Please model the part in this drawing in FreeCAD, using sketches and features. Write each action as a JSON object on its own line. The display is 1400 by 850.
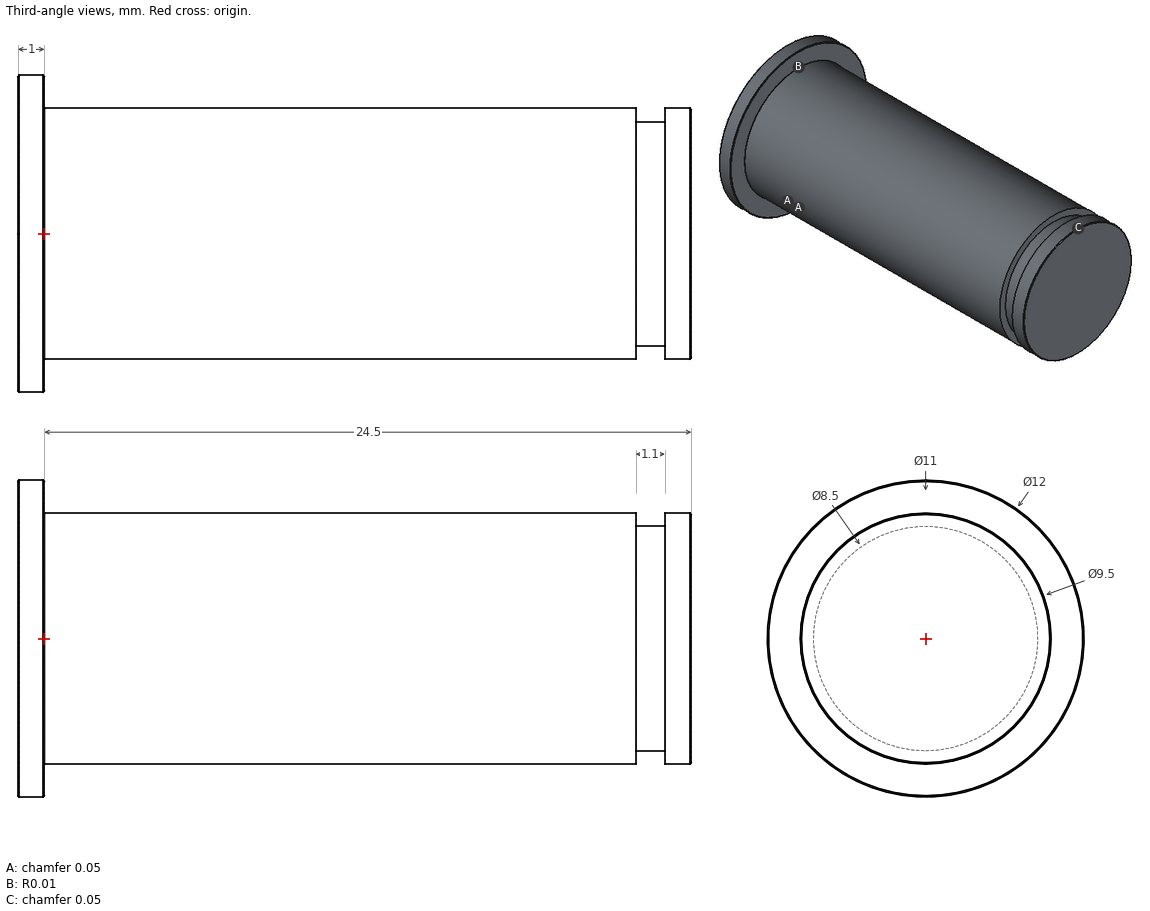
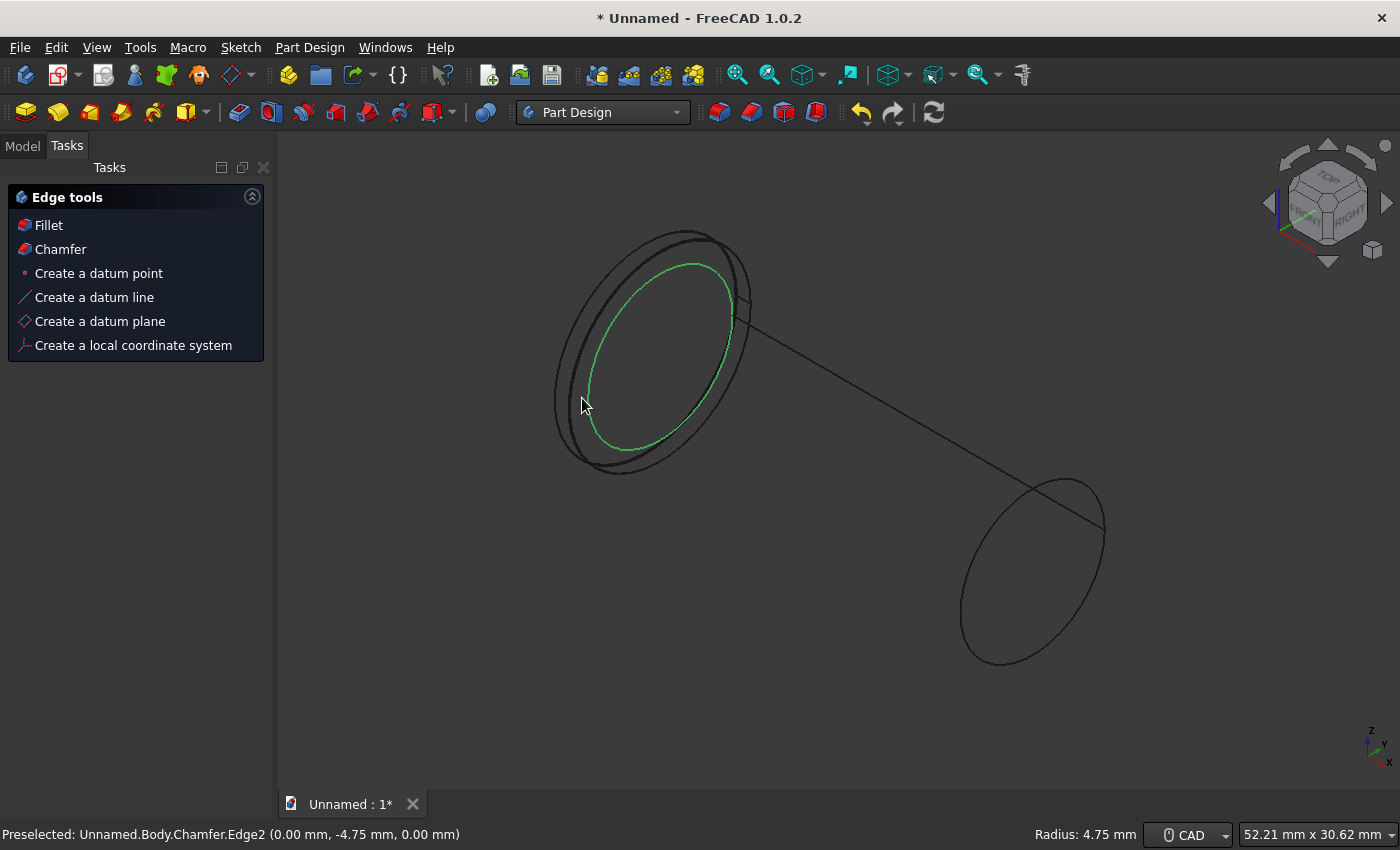
{"action": "key", "text": "v 1"}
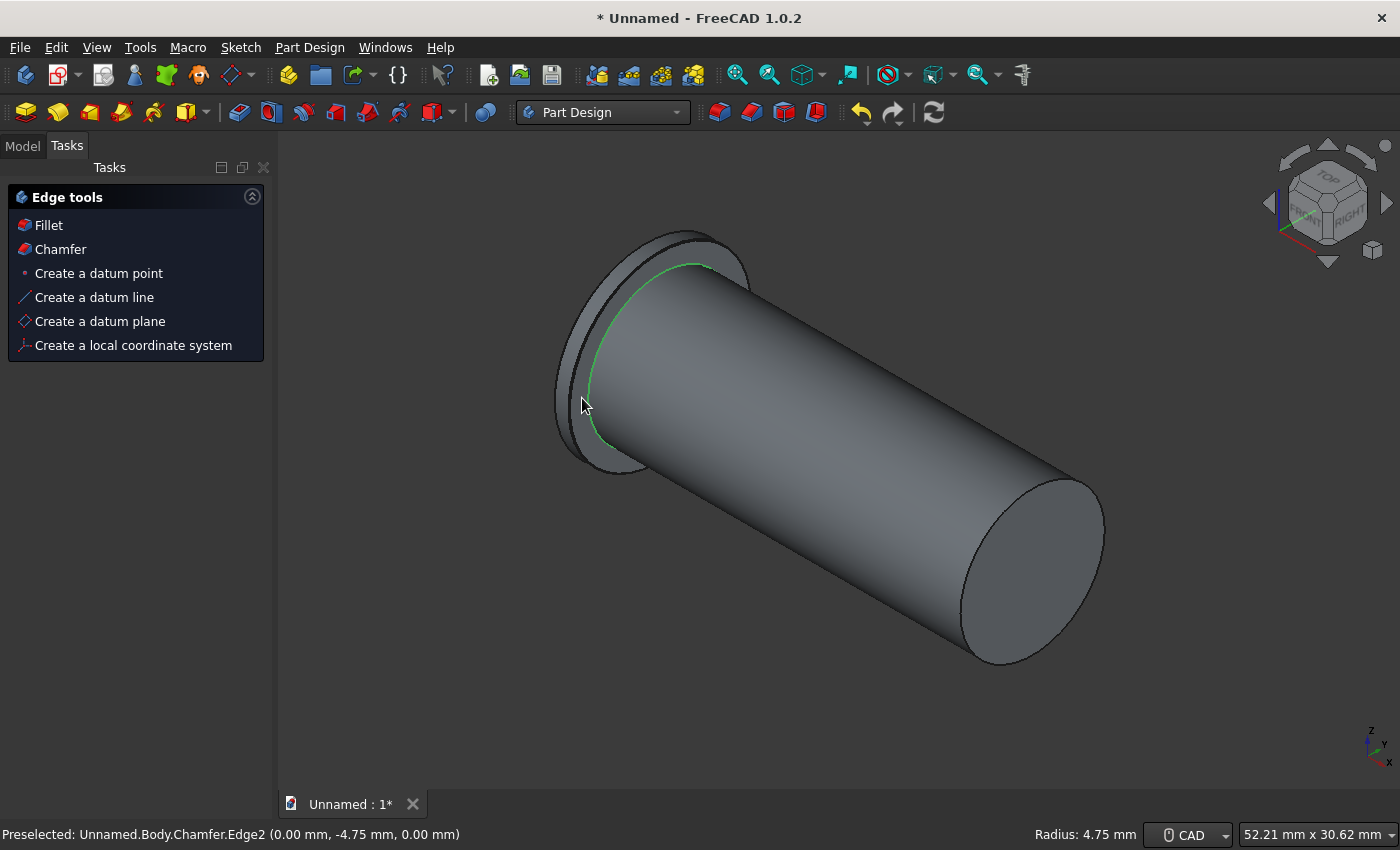
{"action": "left_click", "coordinate": [720, 112]}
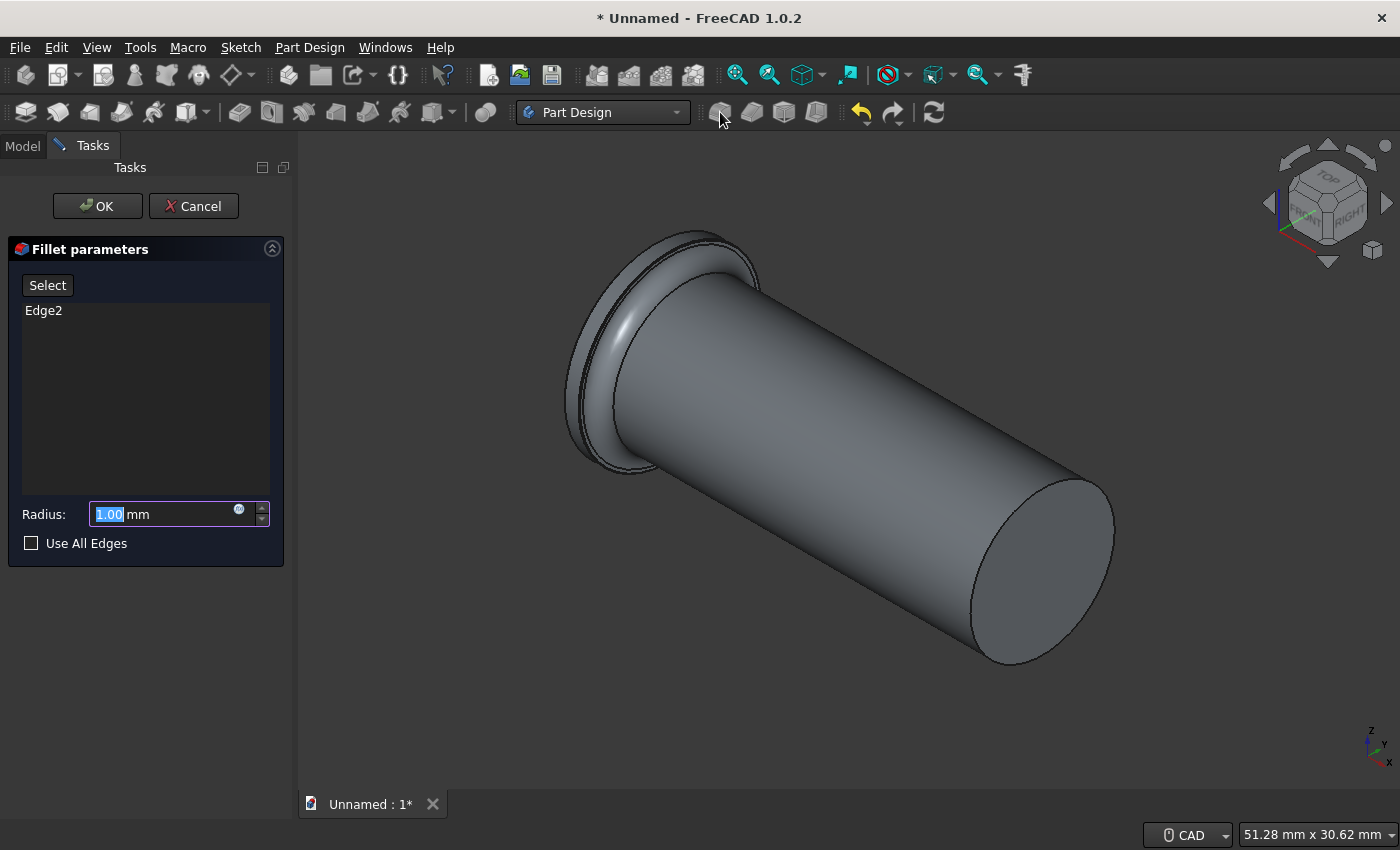
{"action": "type", "text": "0.01"}
{"action": "key", "text": "Tab"}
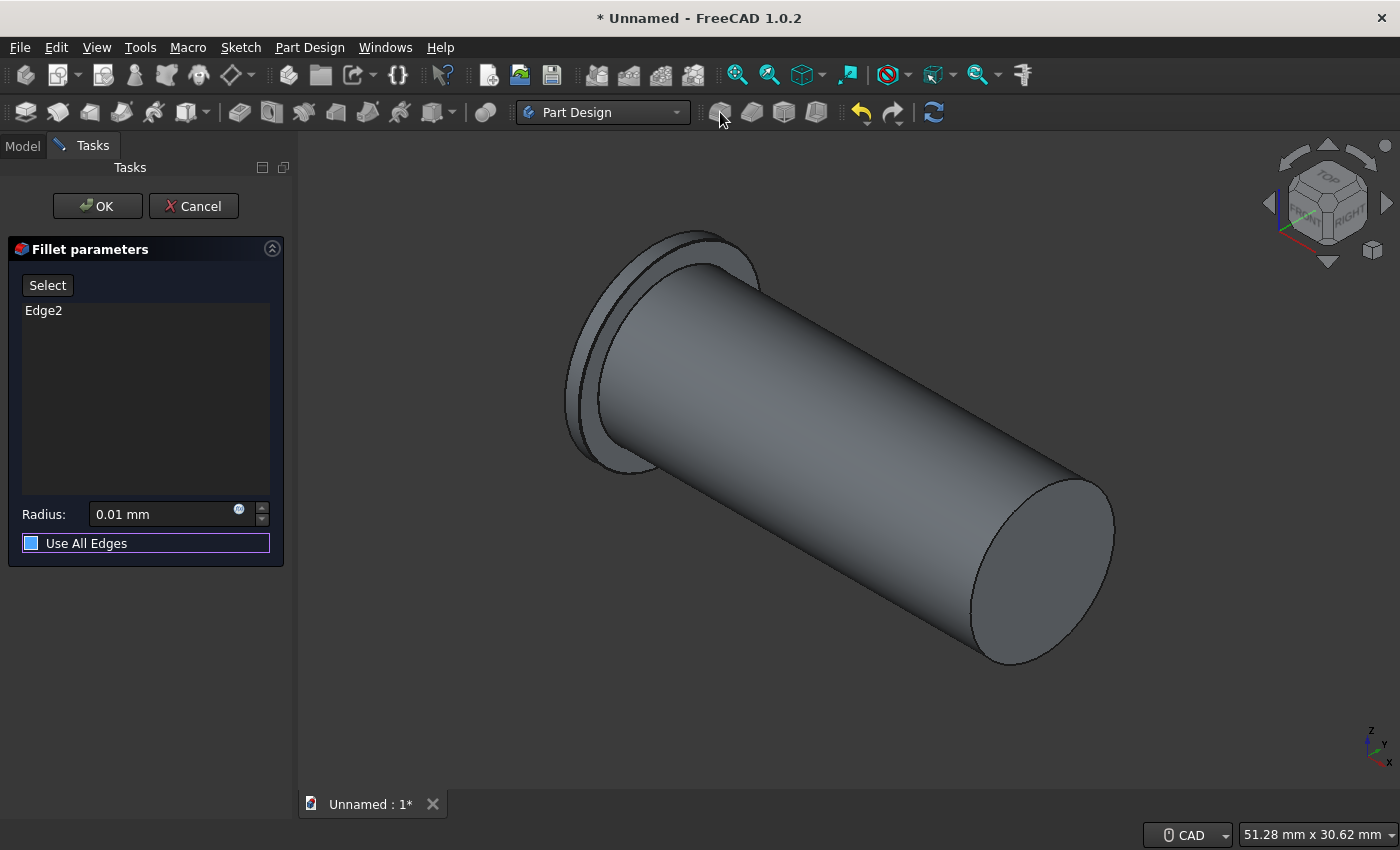
{"action": "left_click", "coordinate": [98, 206]}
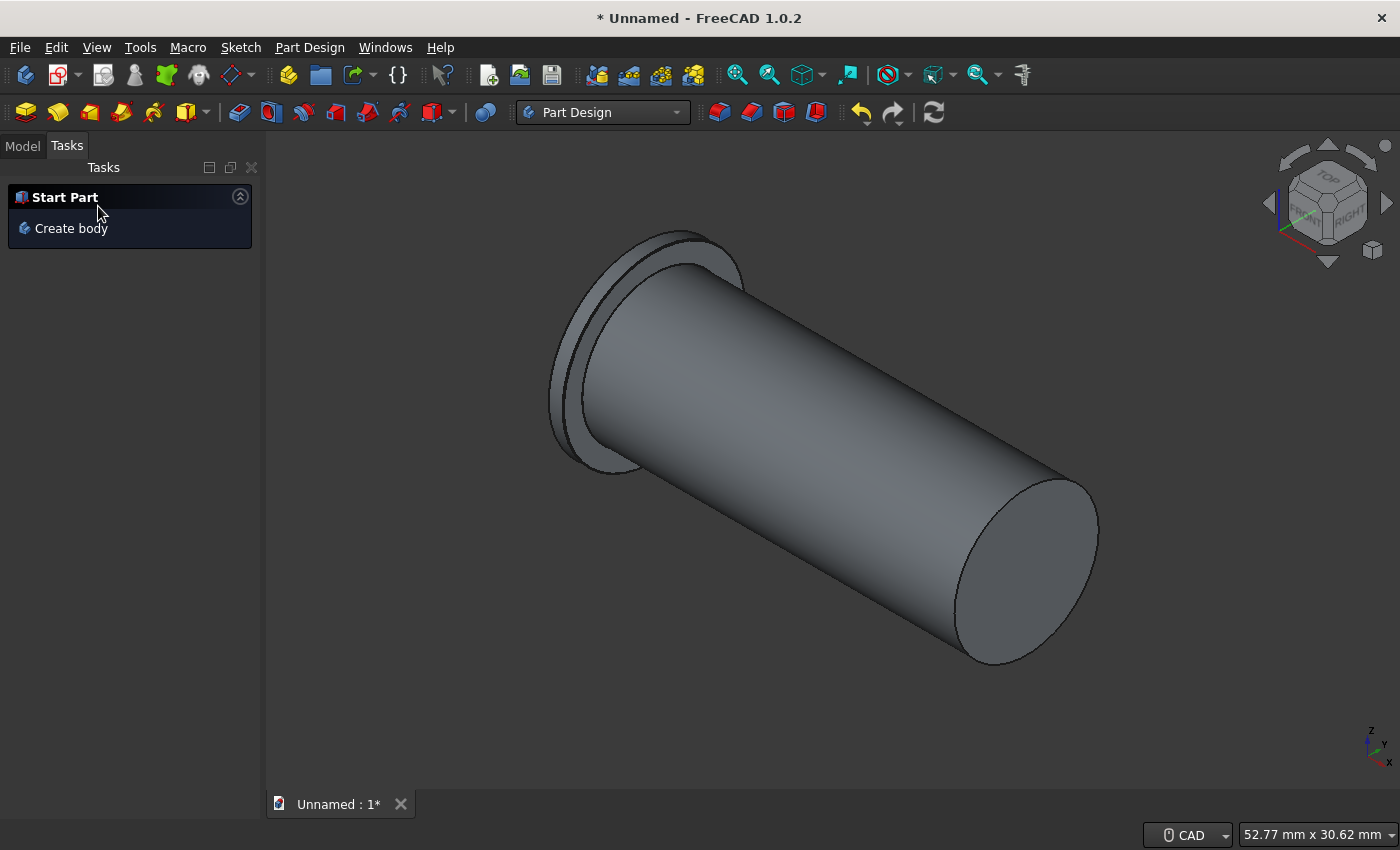
{"action": "left_click", "coordinate": [954, 613]}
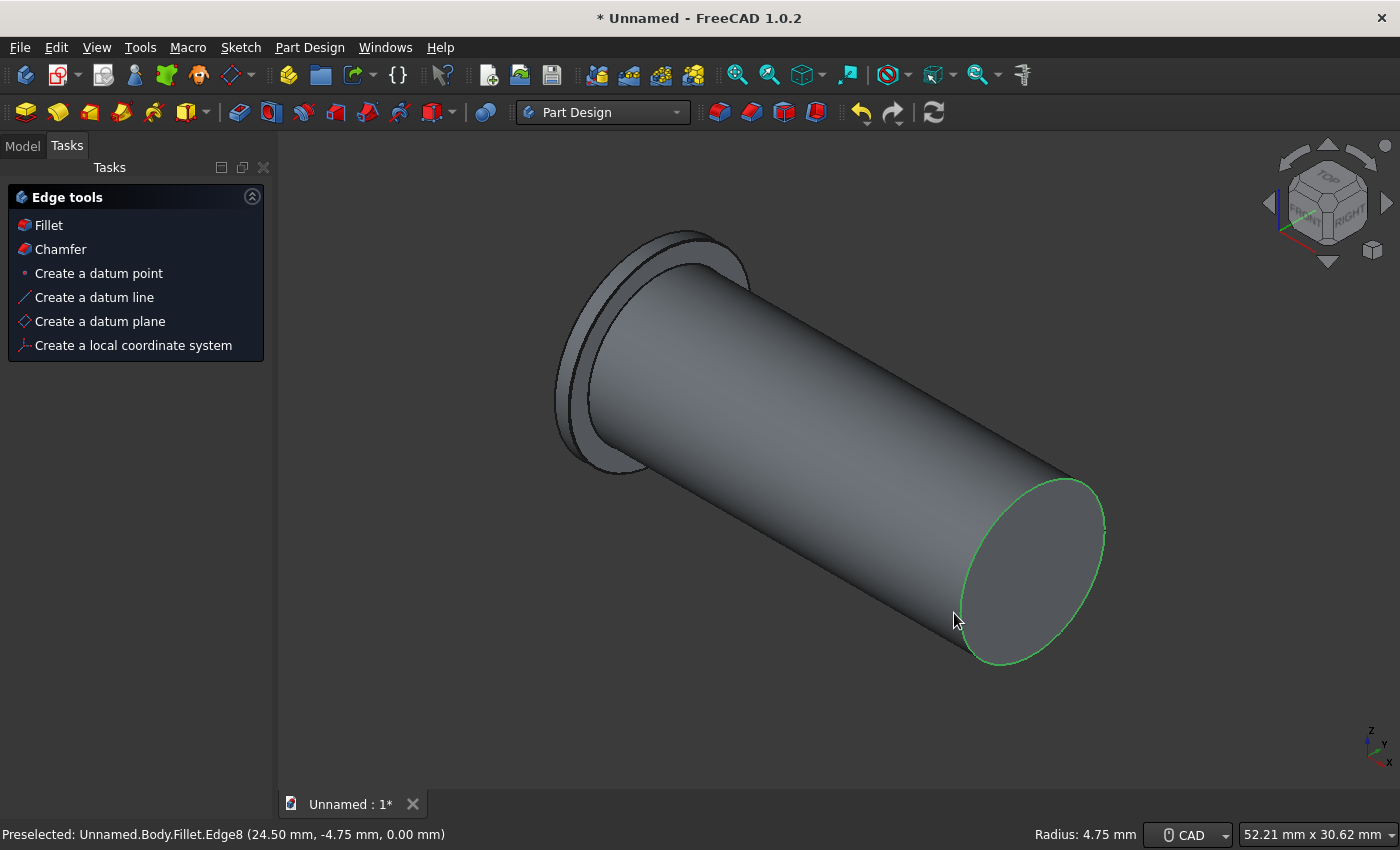
{"action": "left_click", "coordinate": [752, 112]}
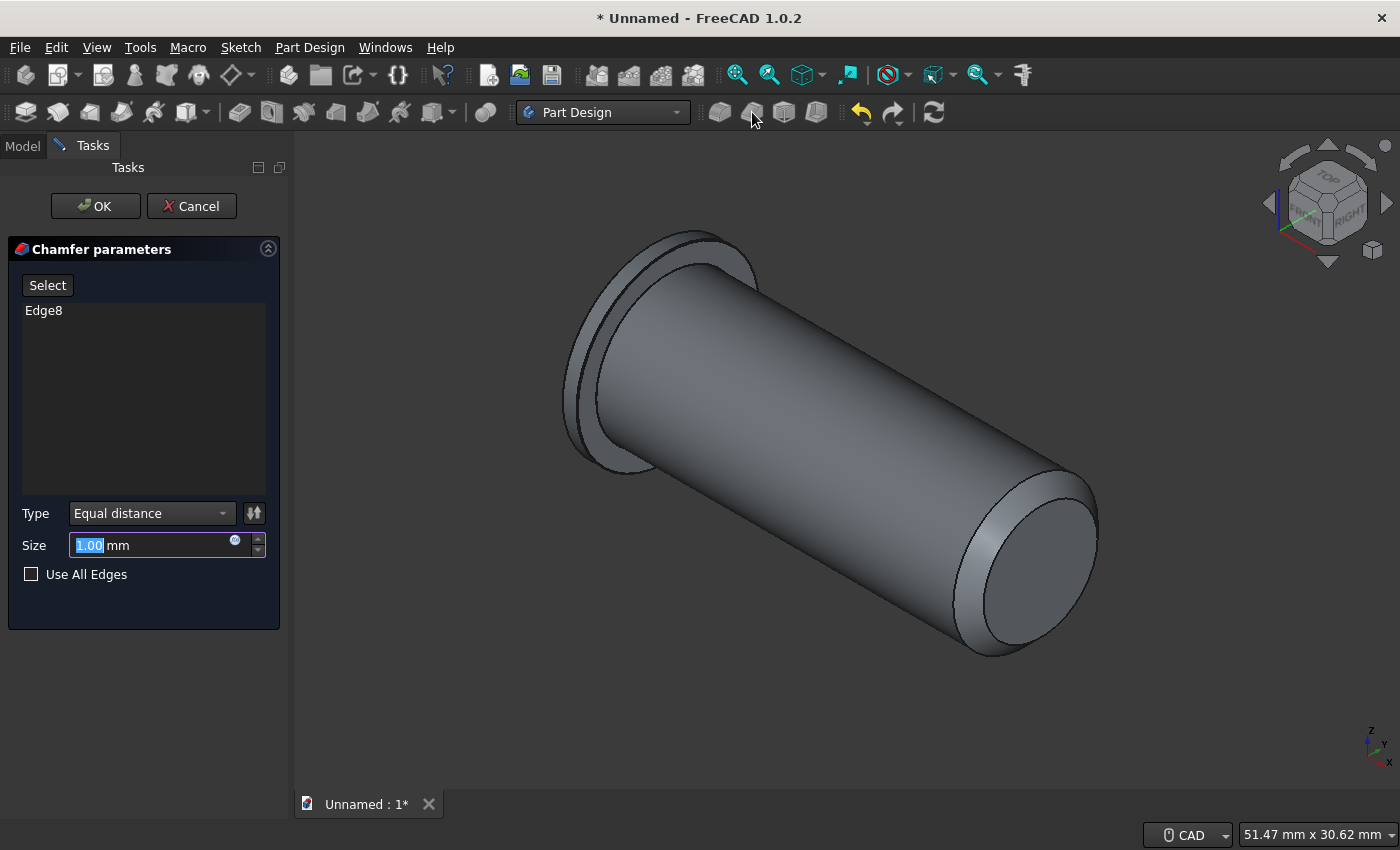
{"action": "type", "text": "0.05"}
{"action": "key", "text": "Tab"}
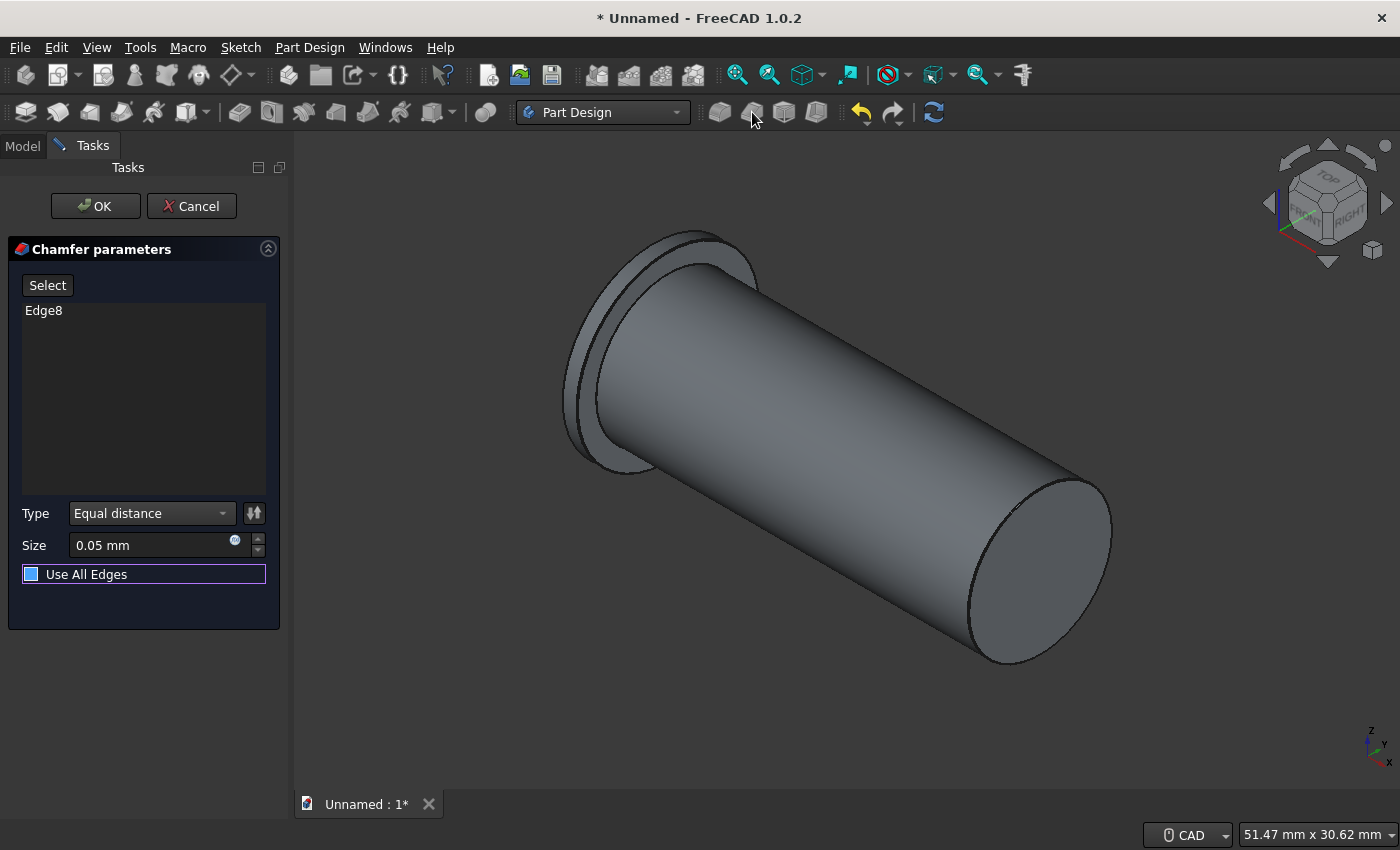
{"action": "left_click", "coordinate": [96, 206]}